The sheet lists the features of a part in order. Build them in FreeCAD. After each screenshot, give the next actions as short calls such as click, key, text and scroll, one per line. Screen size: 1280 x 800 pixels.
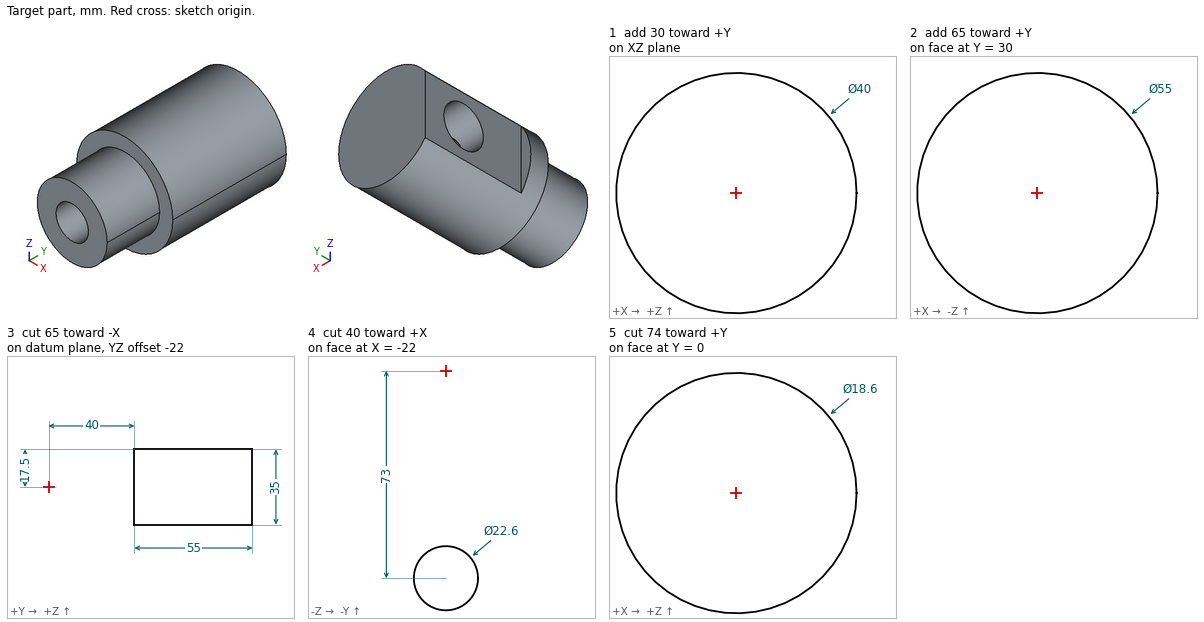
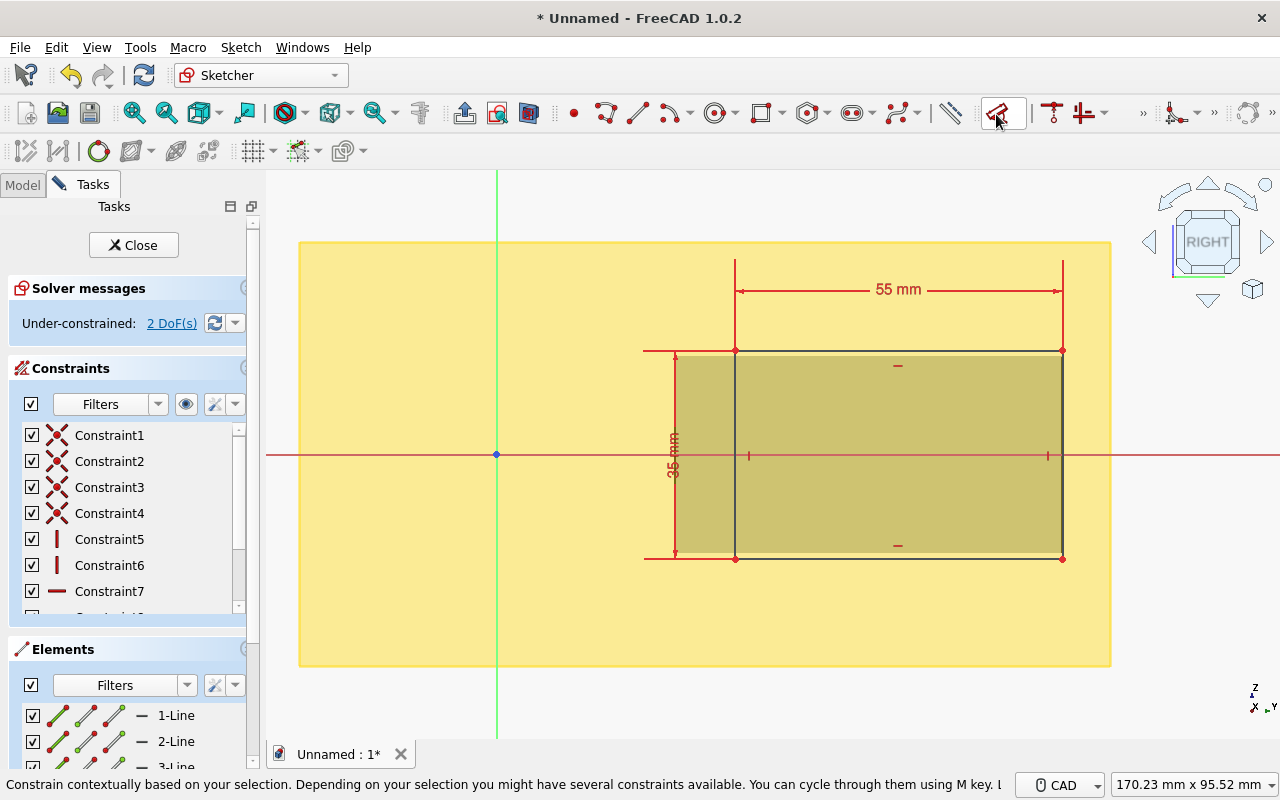
click(735, 351)
click(616, 317)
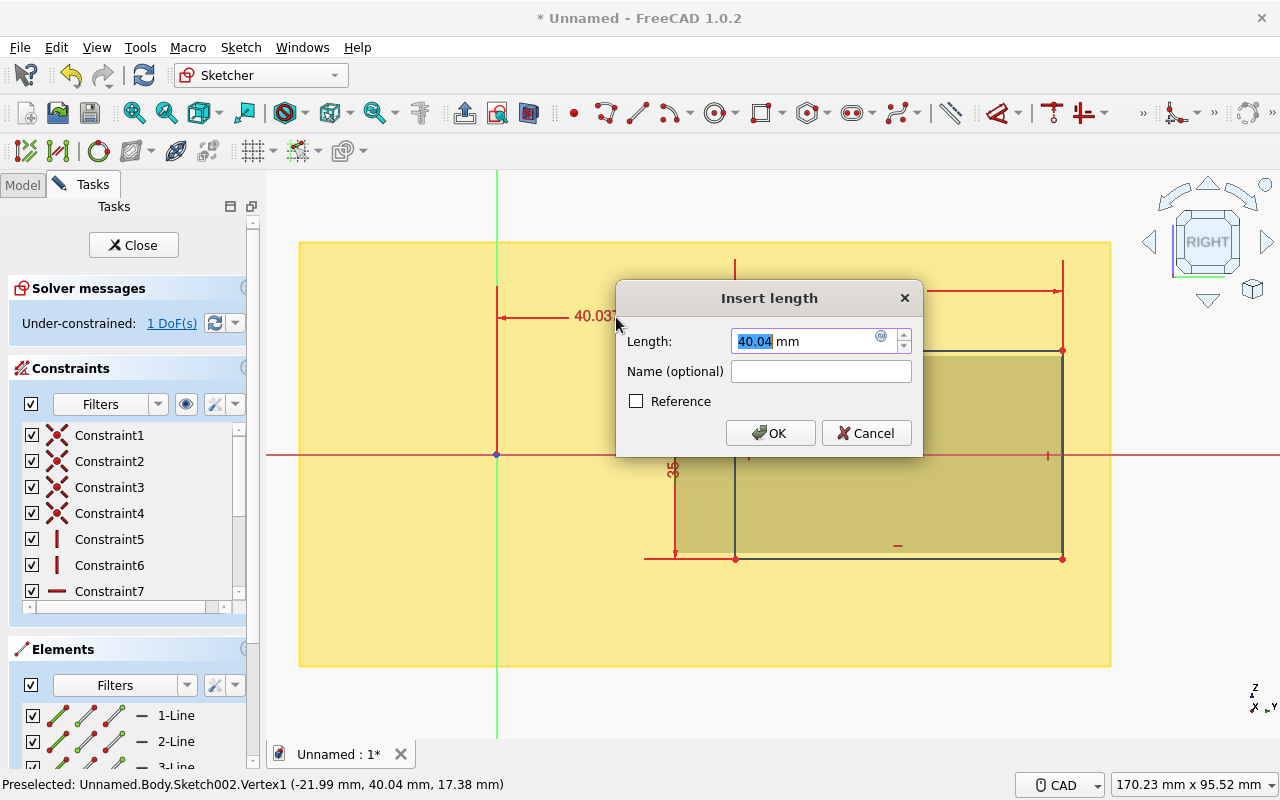
text(40)
key(Return)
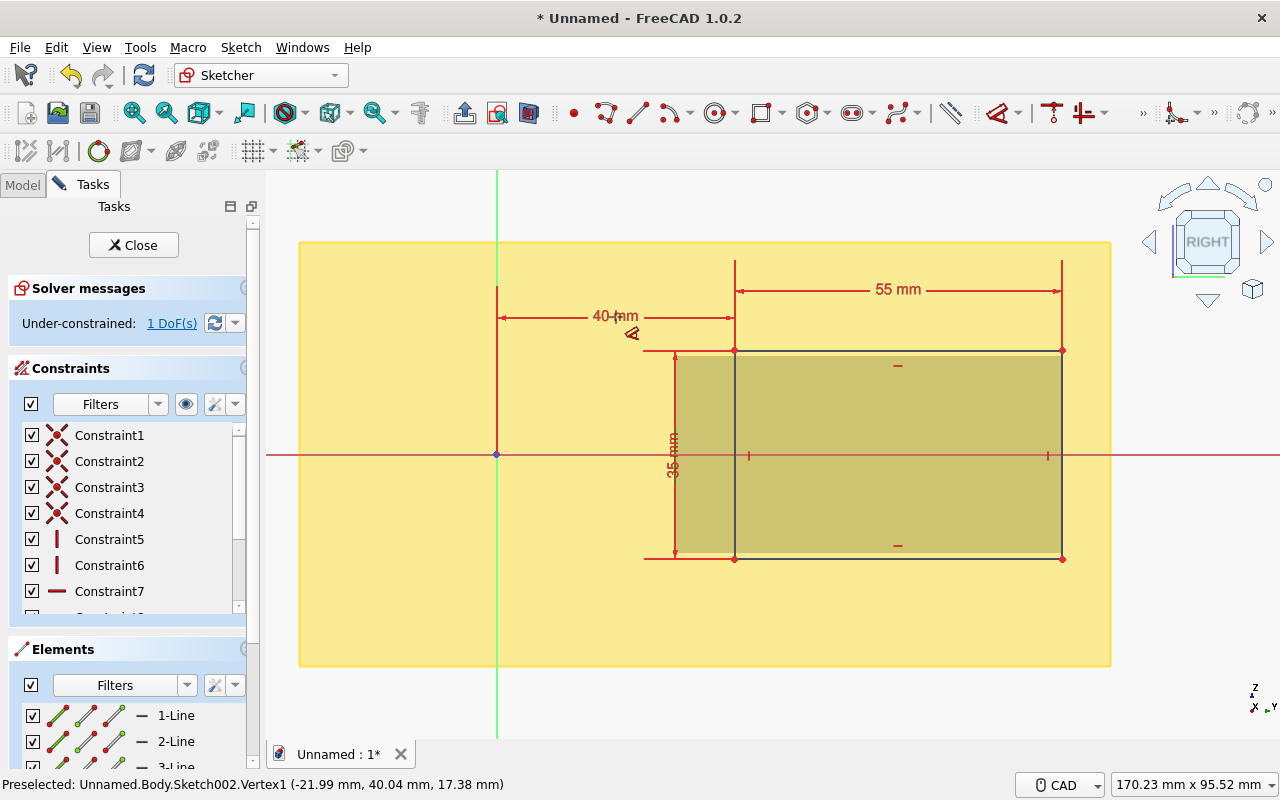
click(735, 351)
click(463, 403)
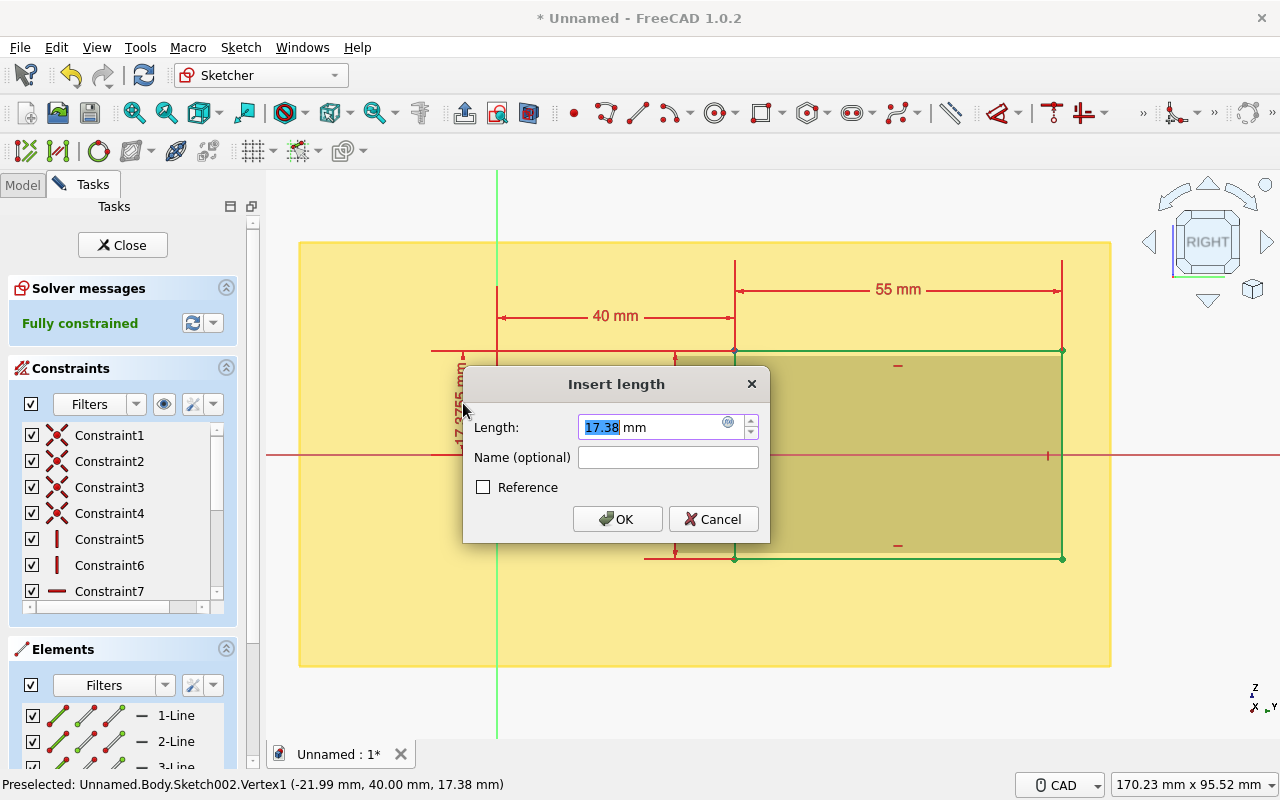
text(17.5)
key(Return)
key(Escape)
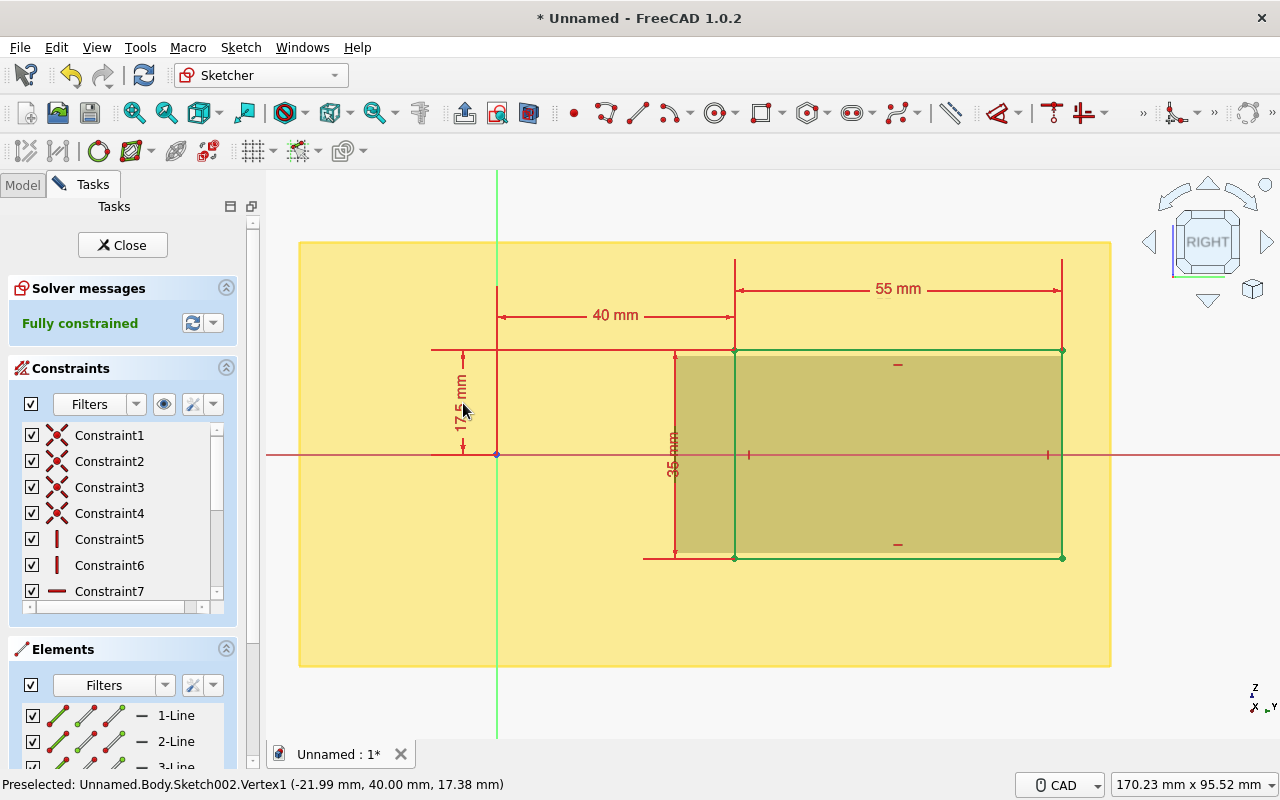
click(123, 245)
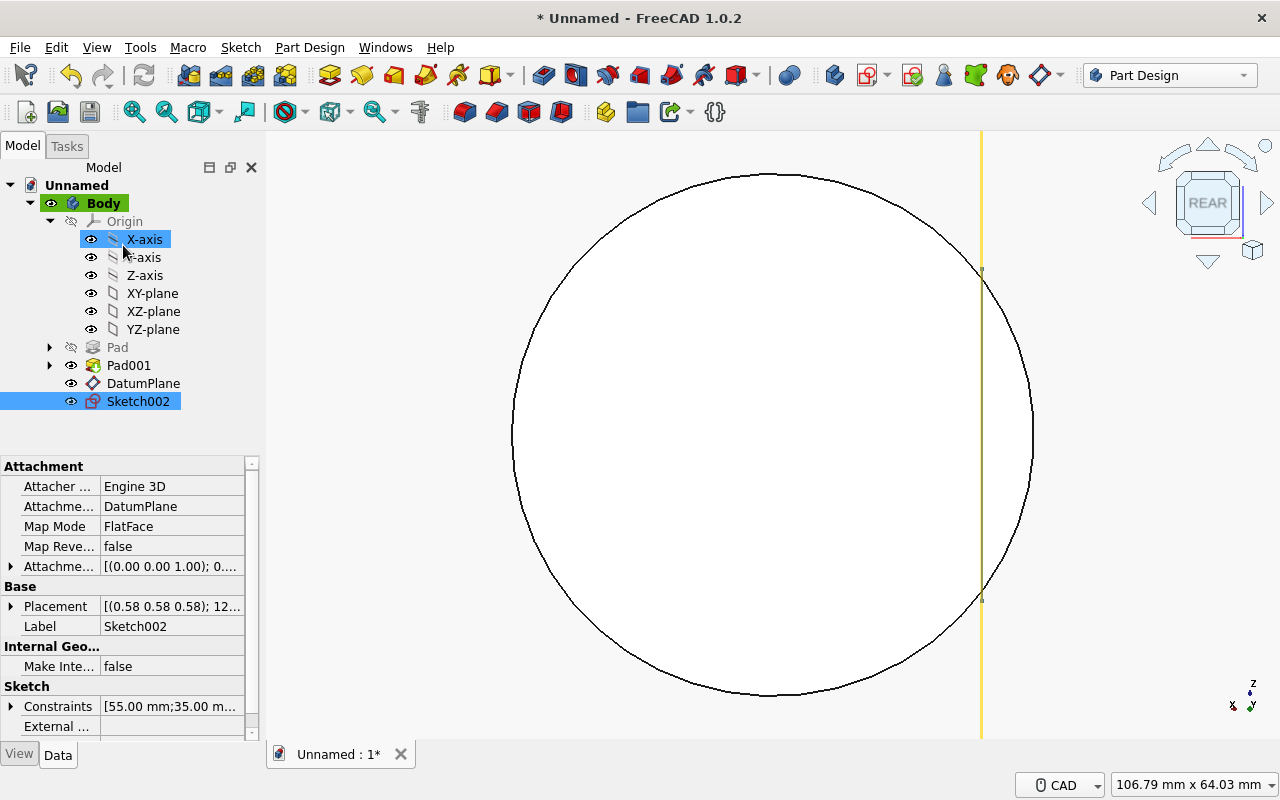
click(544, 76)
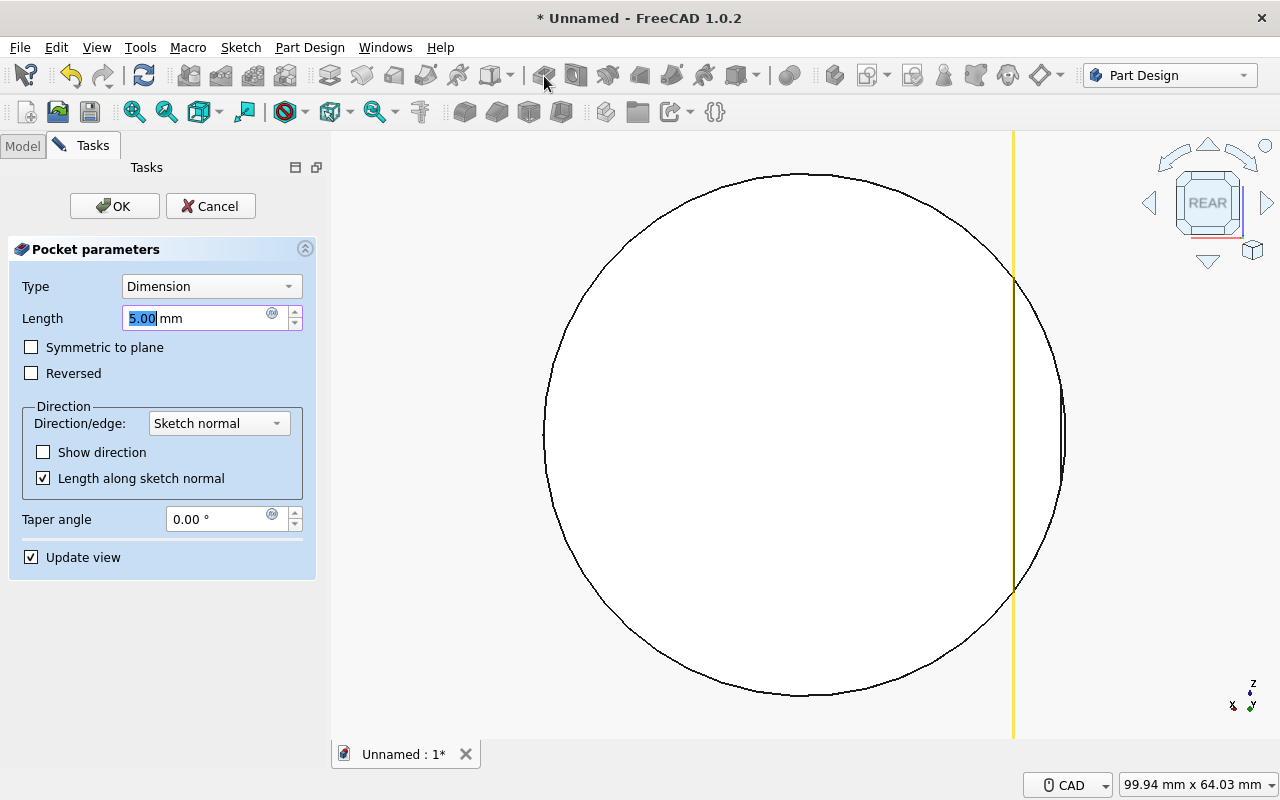
text(65)
key(Tab)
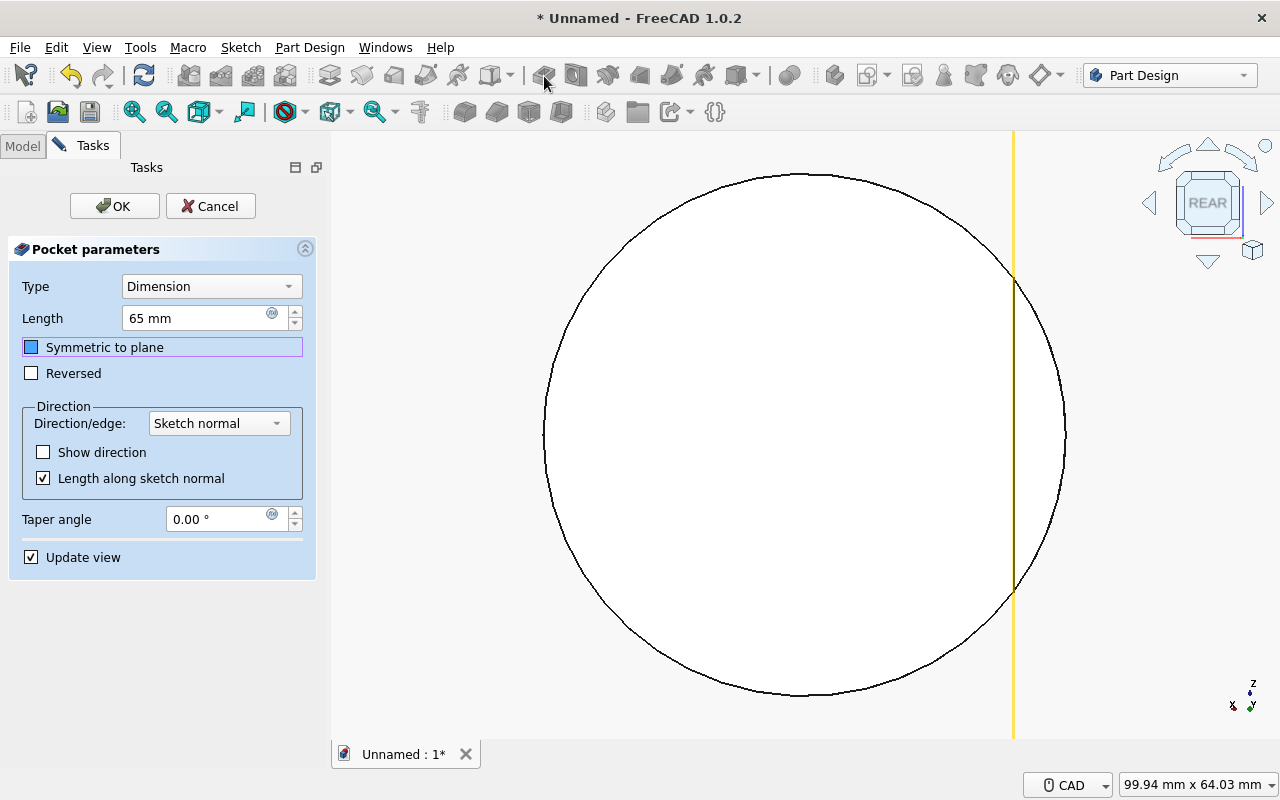
click(115, 206)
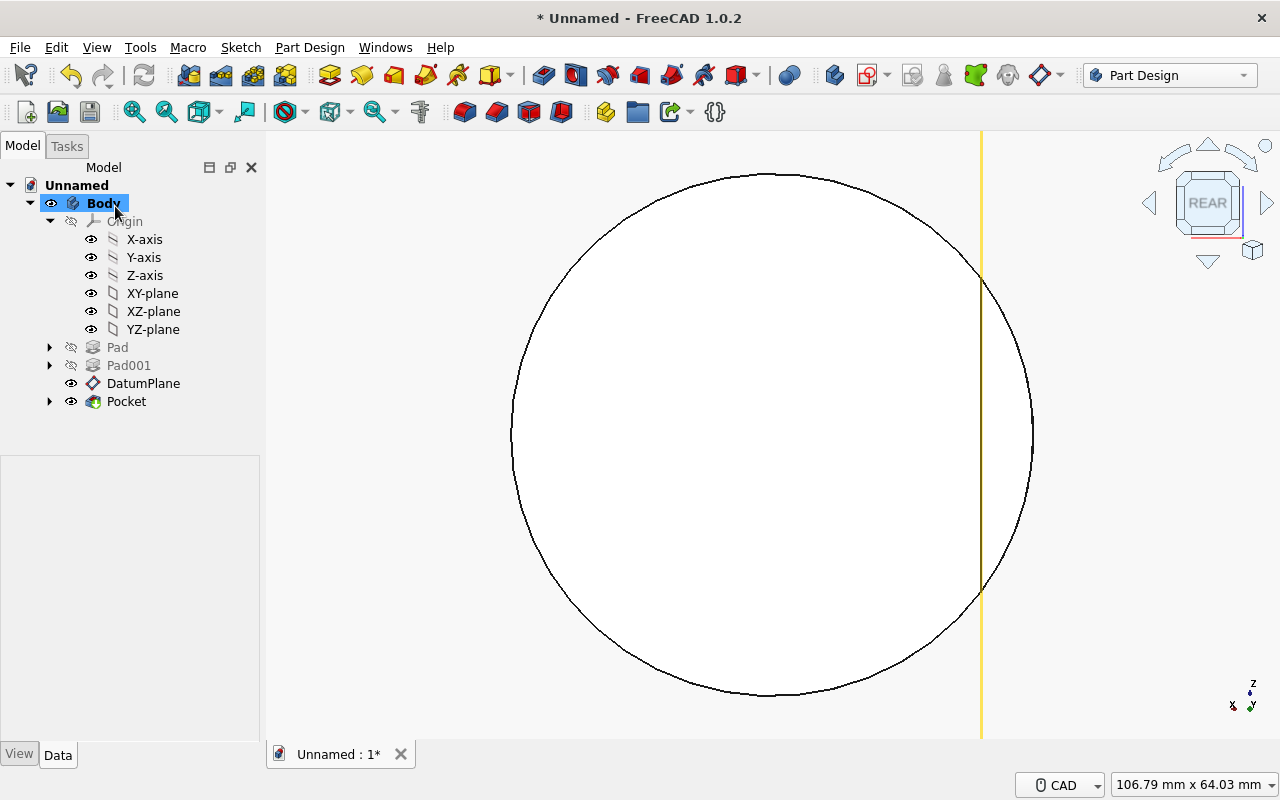
click(116, 383)
key(space)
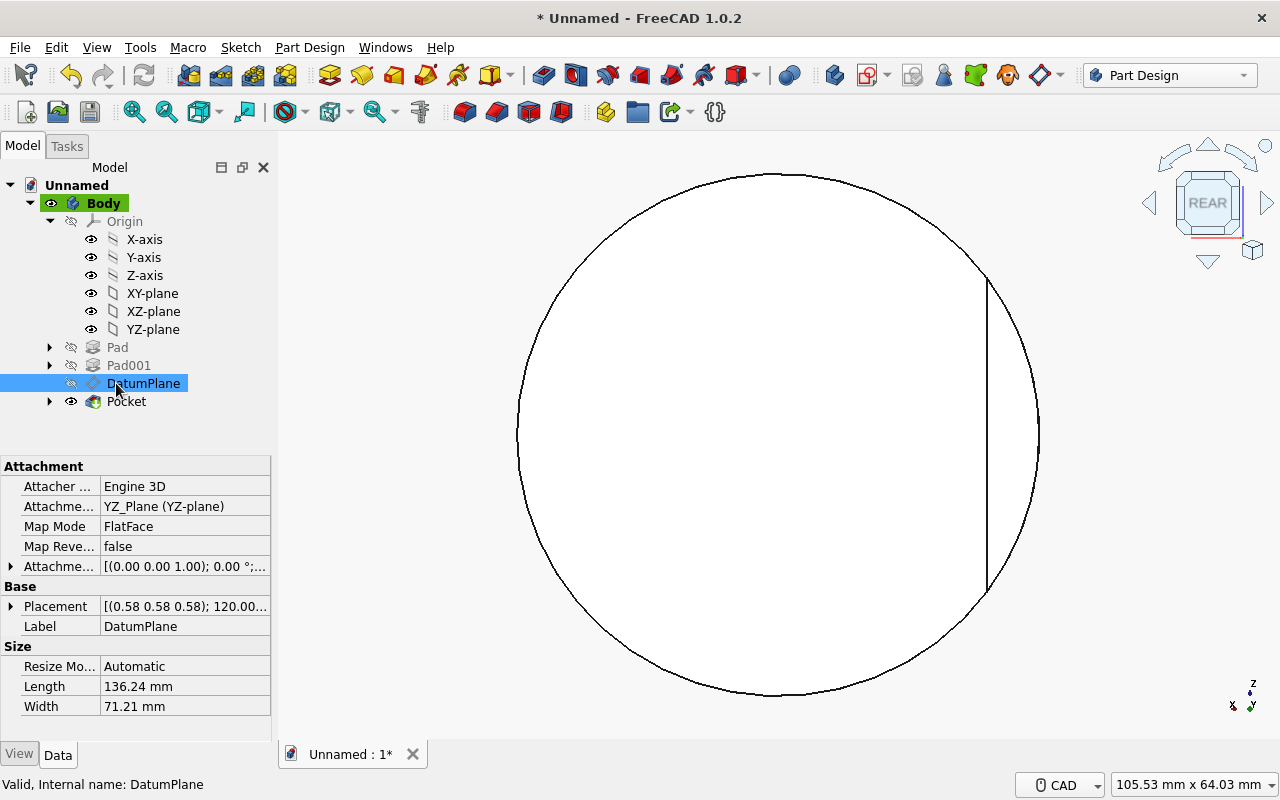
key(6)